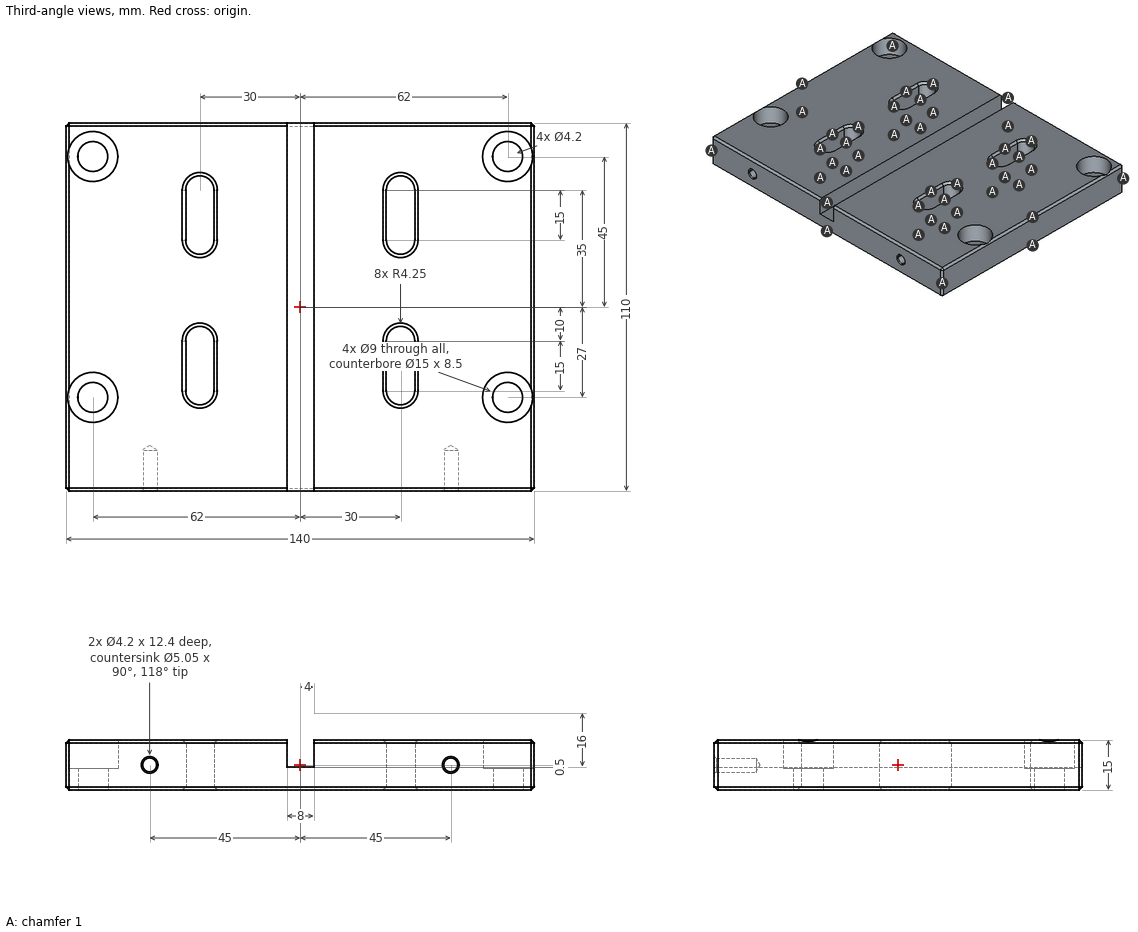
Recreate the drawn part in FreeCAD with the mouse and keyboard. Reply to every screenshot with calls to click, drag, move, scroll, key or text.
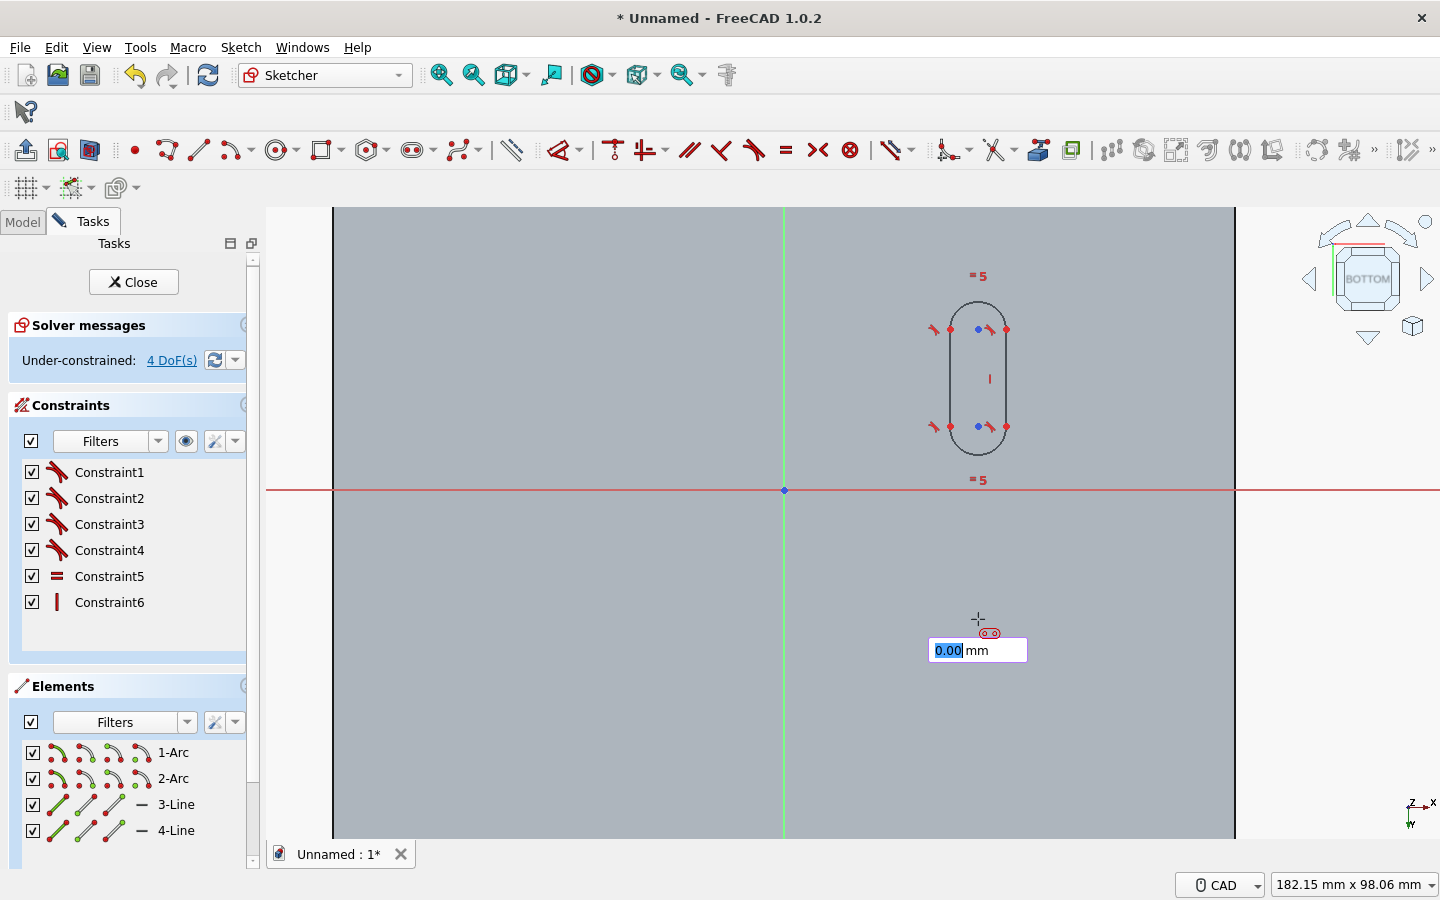
click(950, 668)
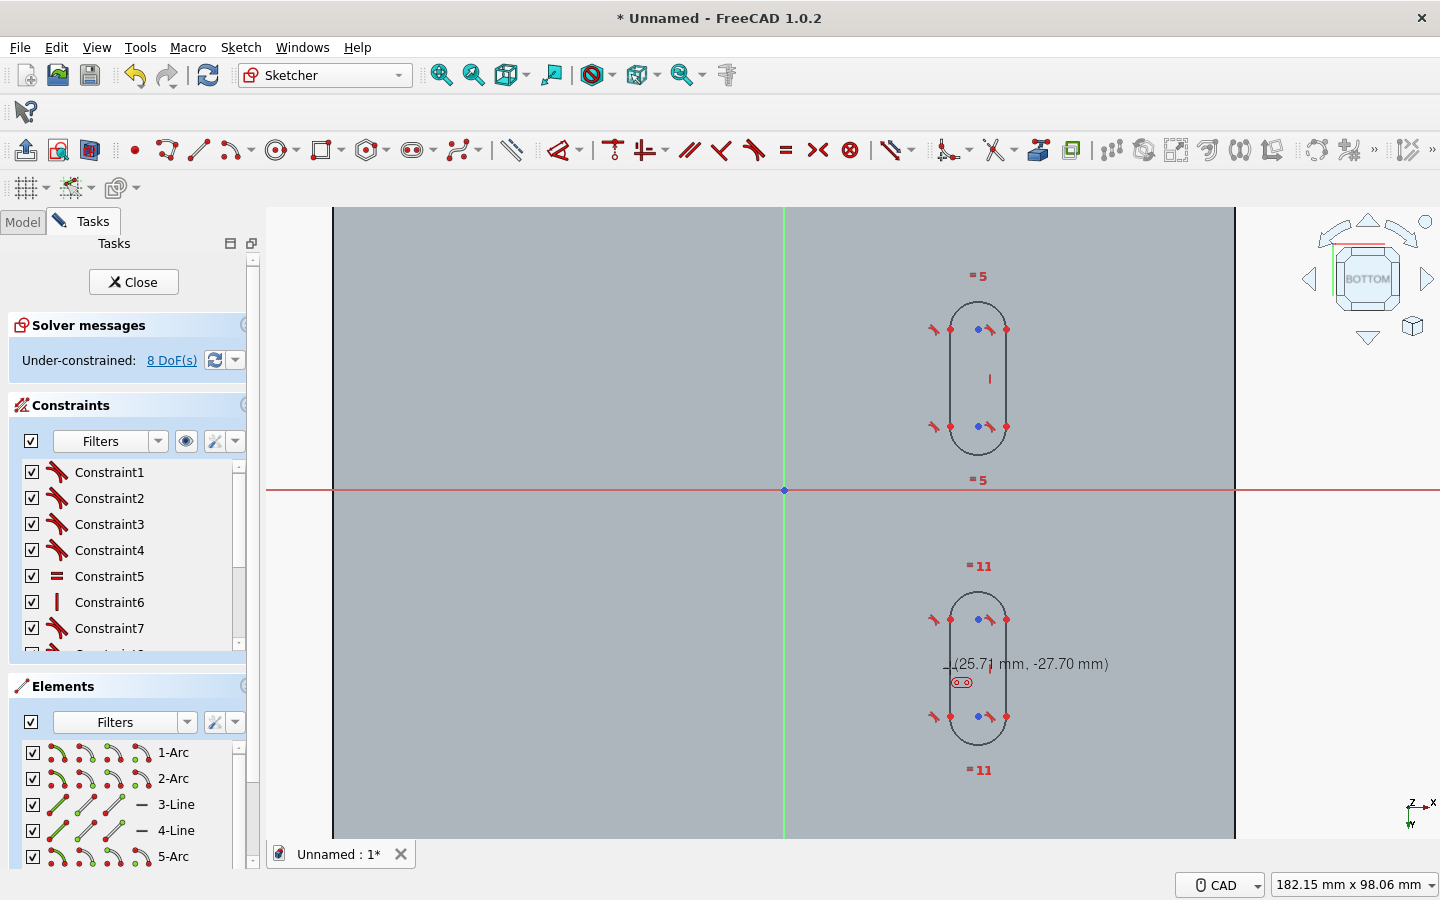
click(591, 716)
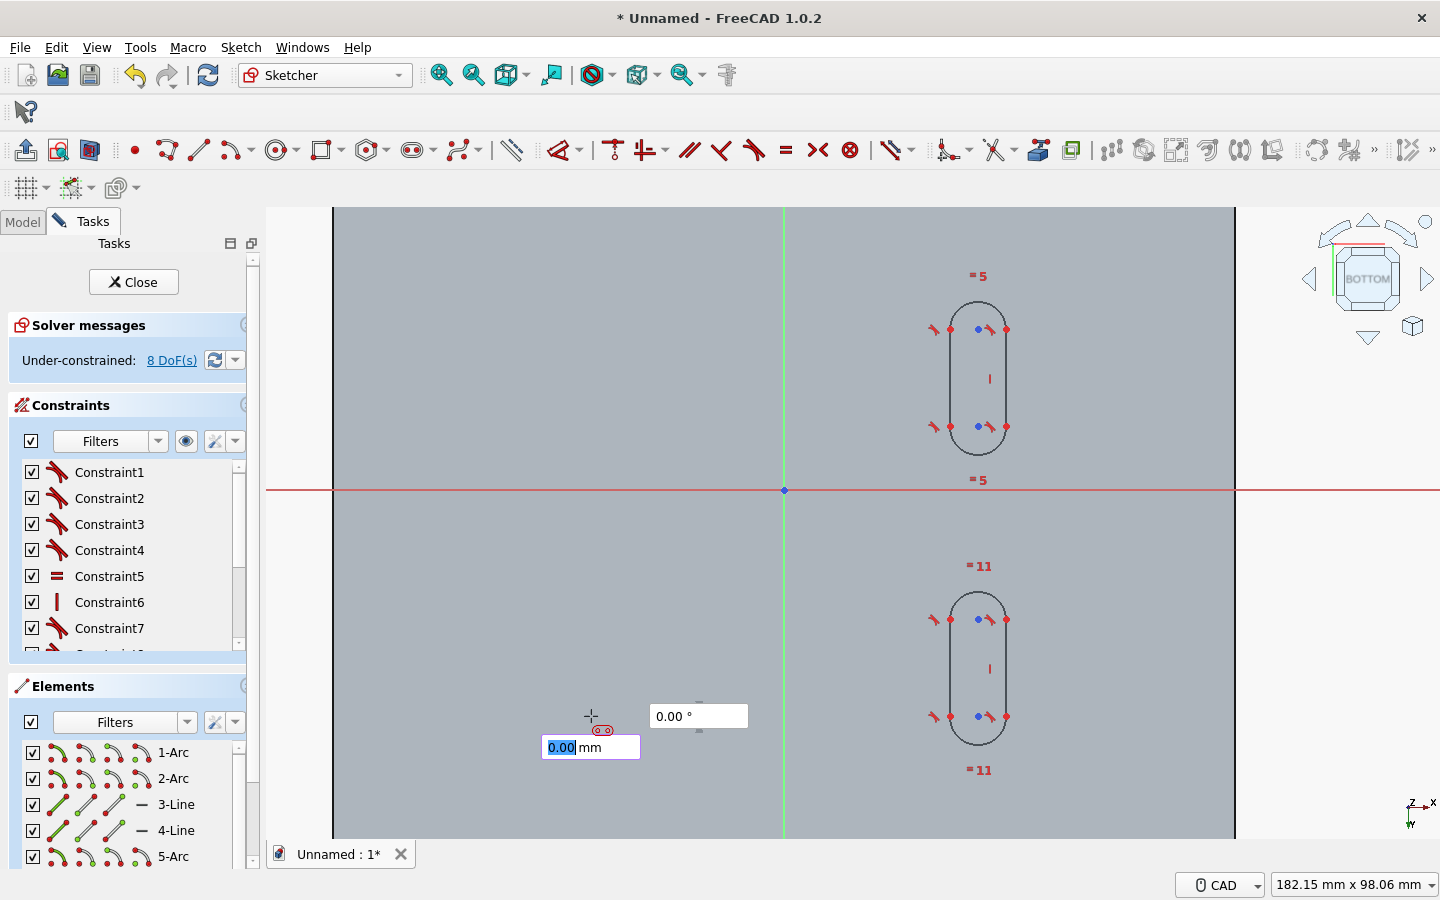
click(591, 619)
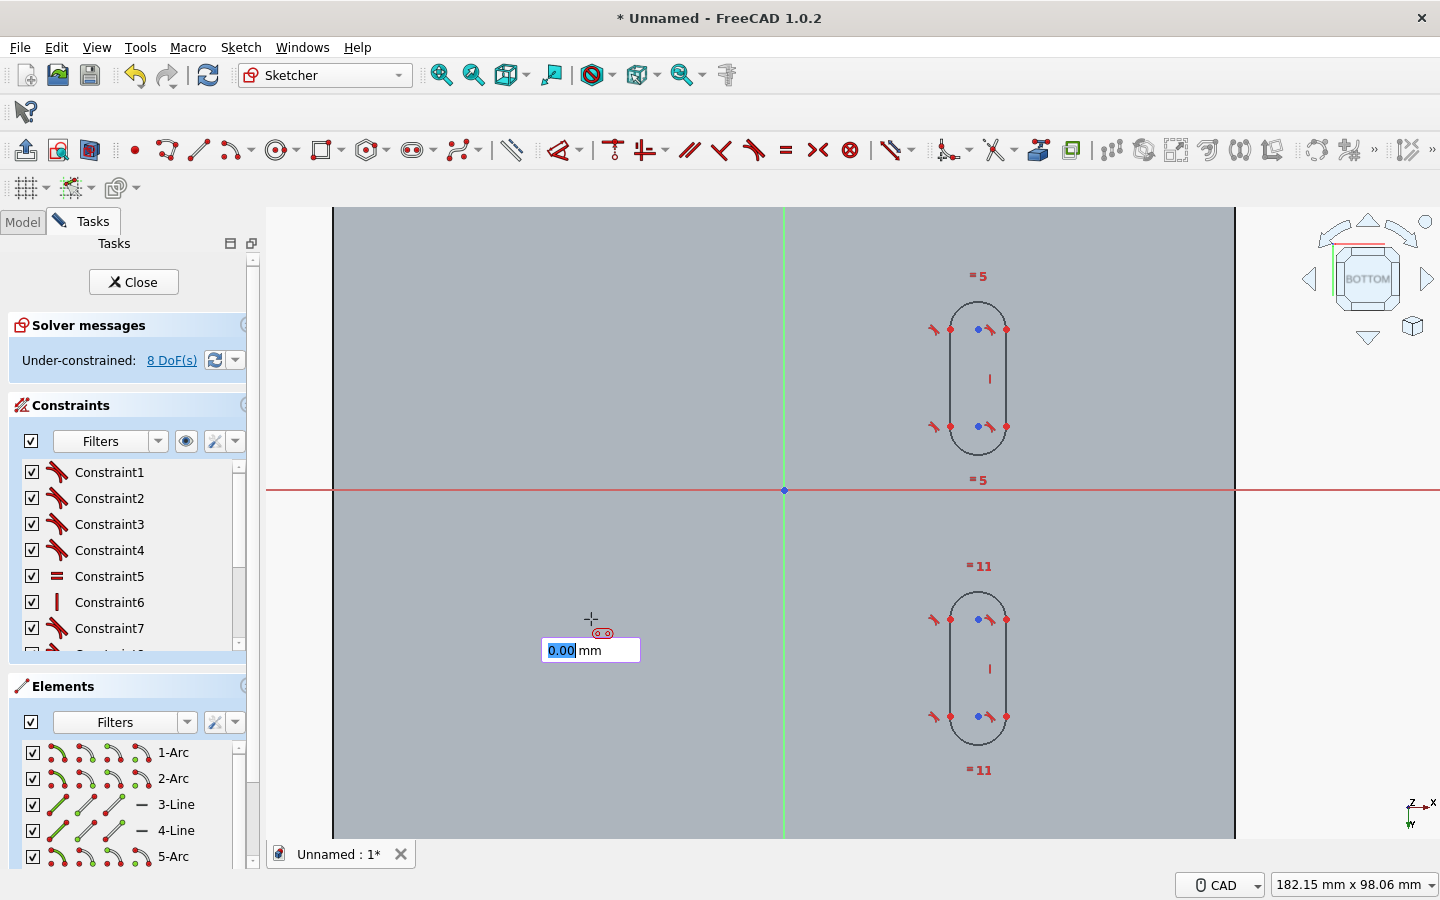
click(618, 668)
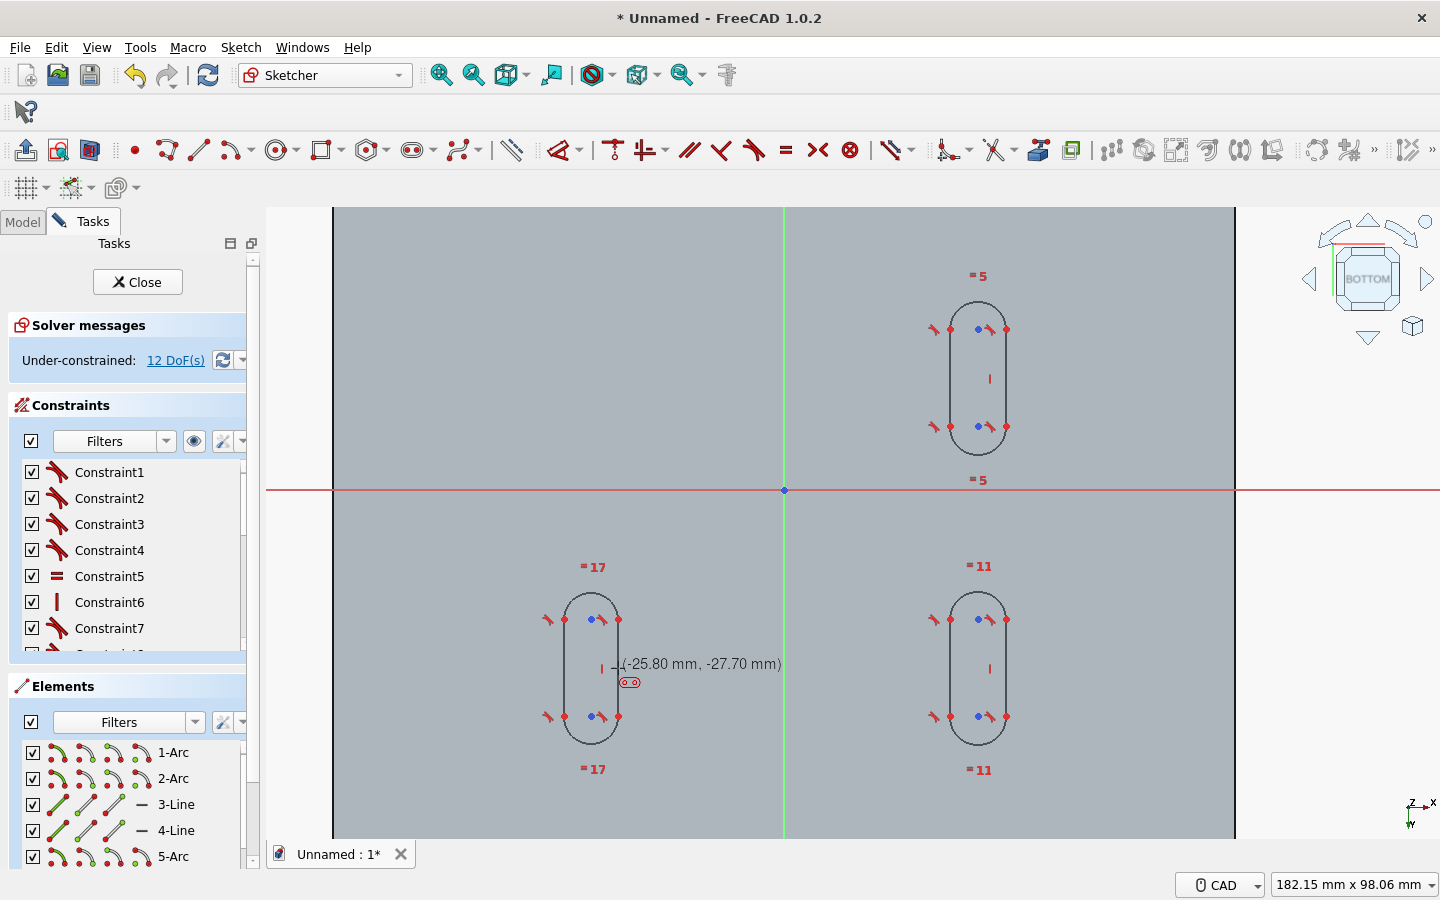
click(591, 426)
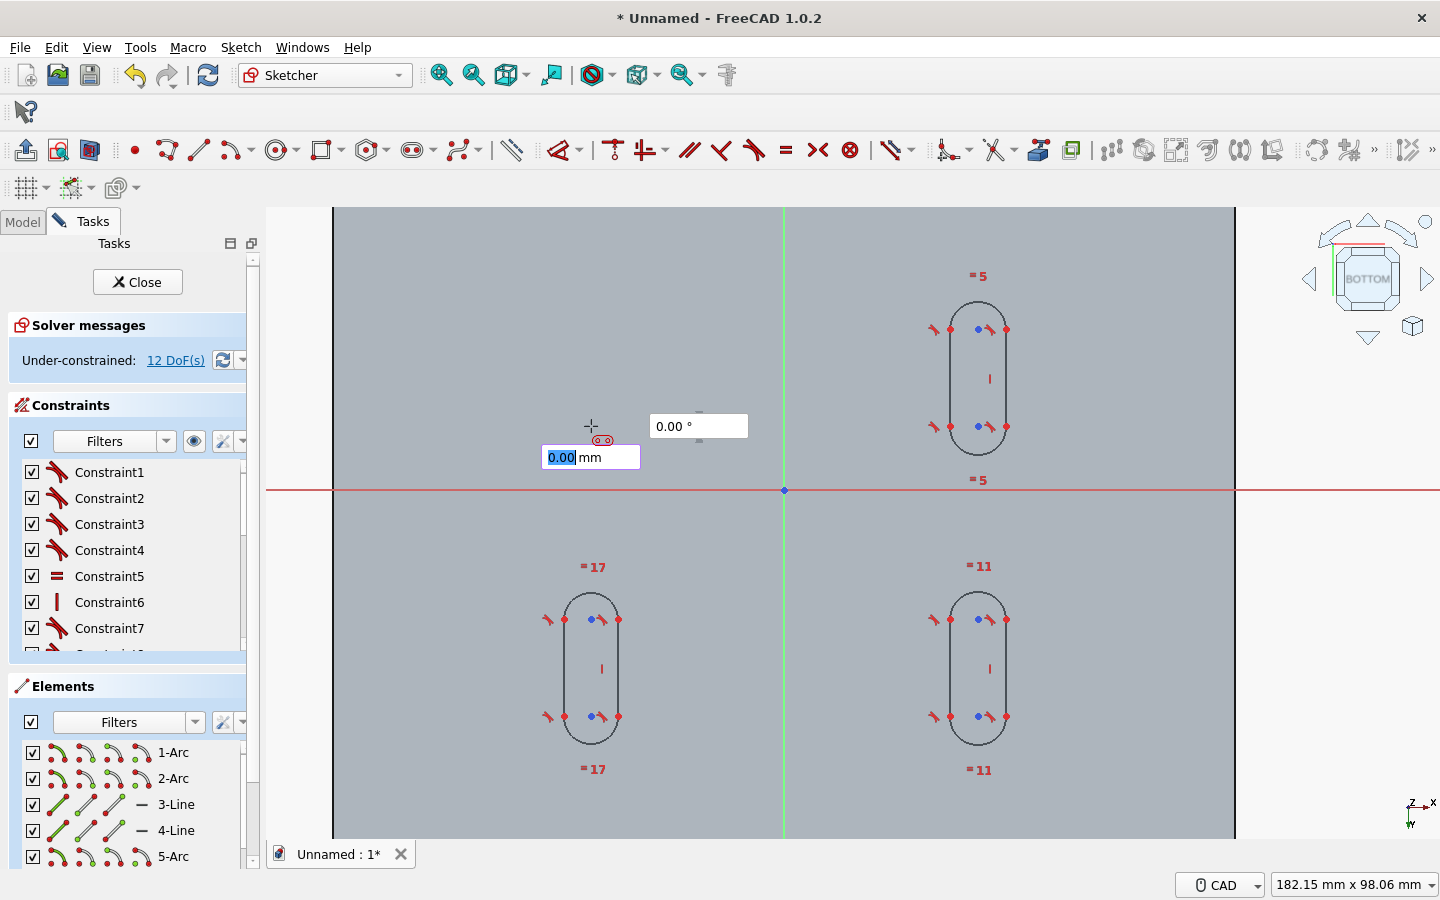
click(591, 329)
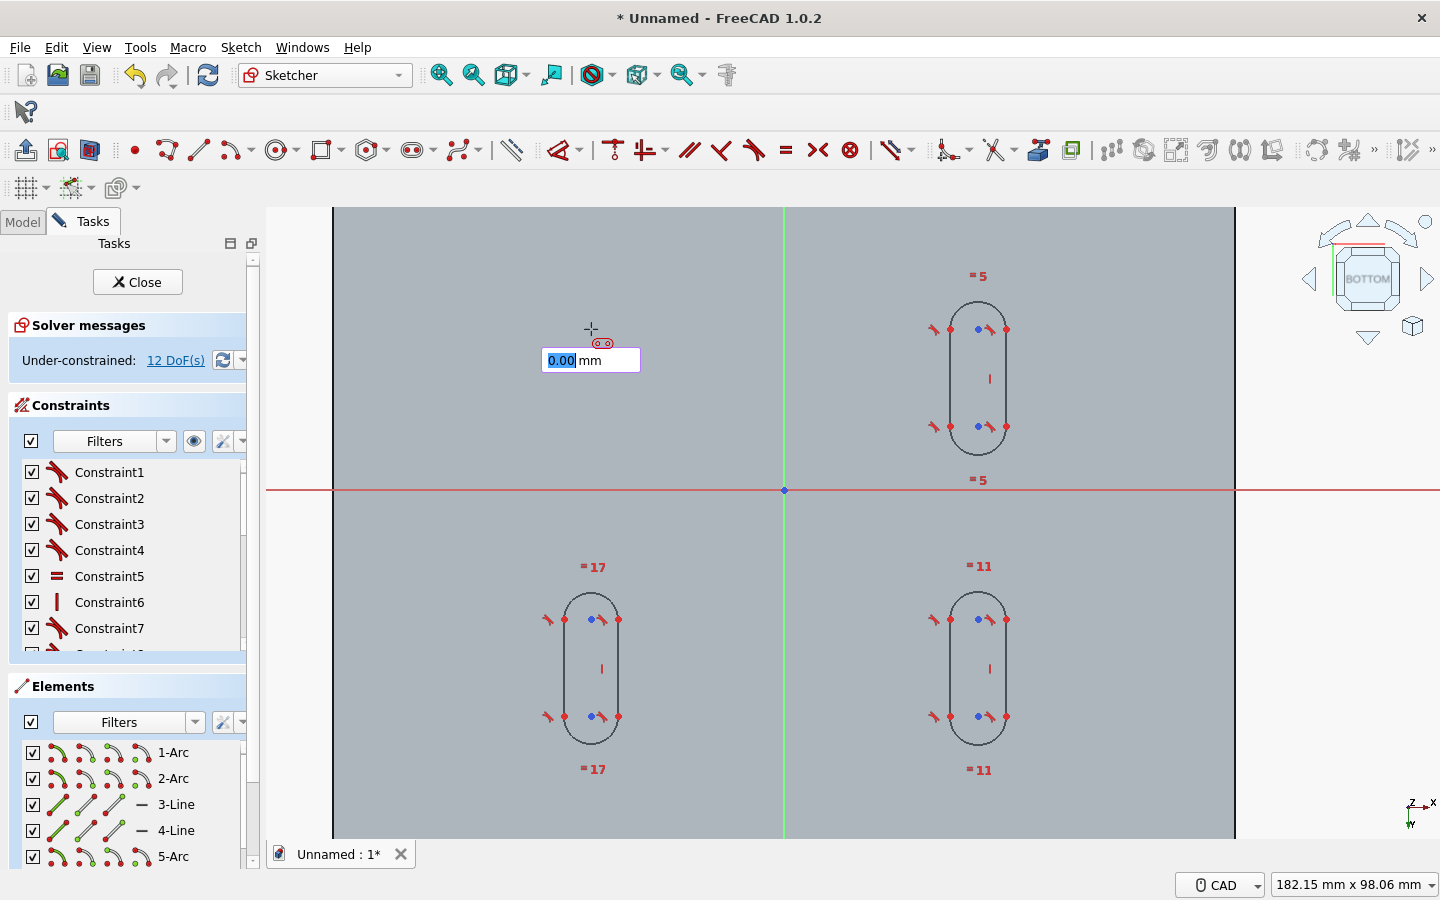
click(618, 378)
key(Escape)